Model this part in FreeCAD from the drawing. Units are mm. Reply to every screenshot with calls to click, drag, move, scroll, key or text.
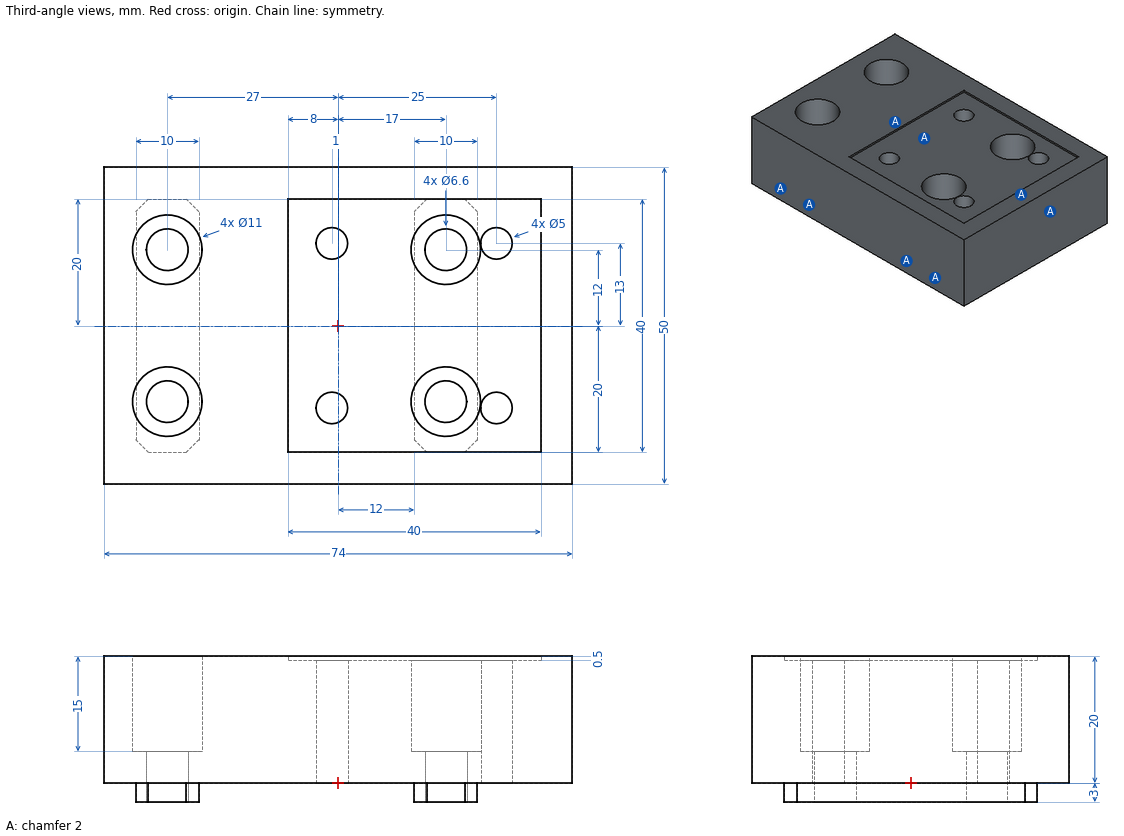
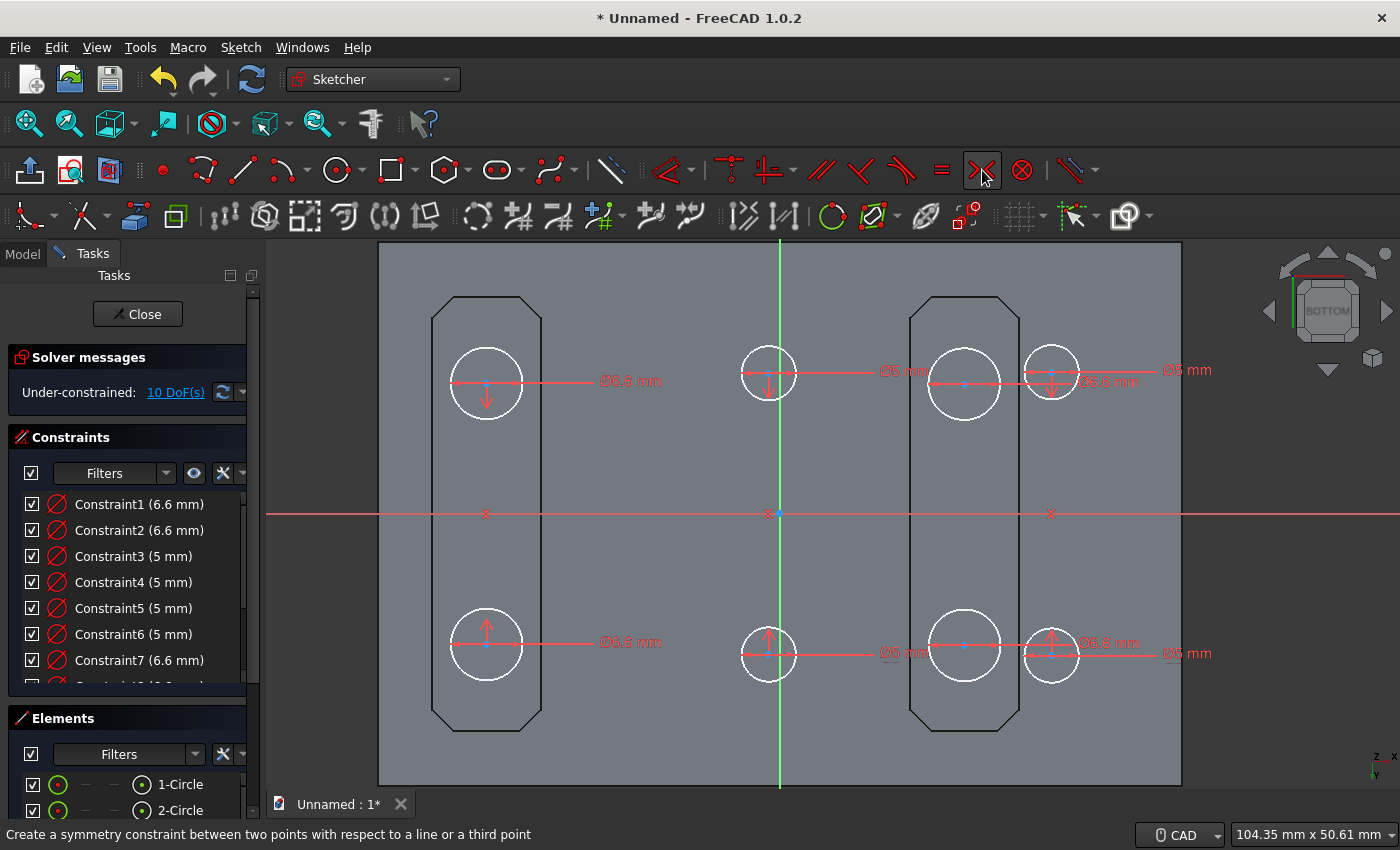
click(965, 645)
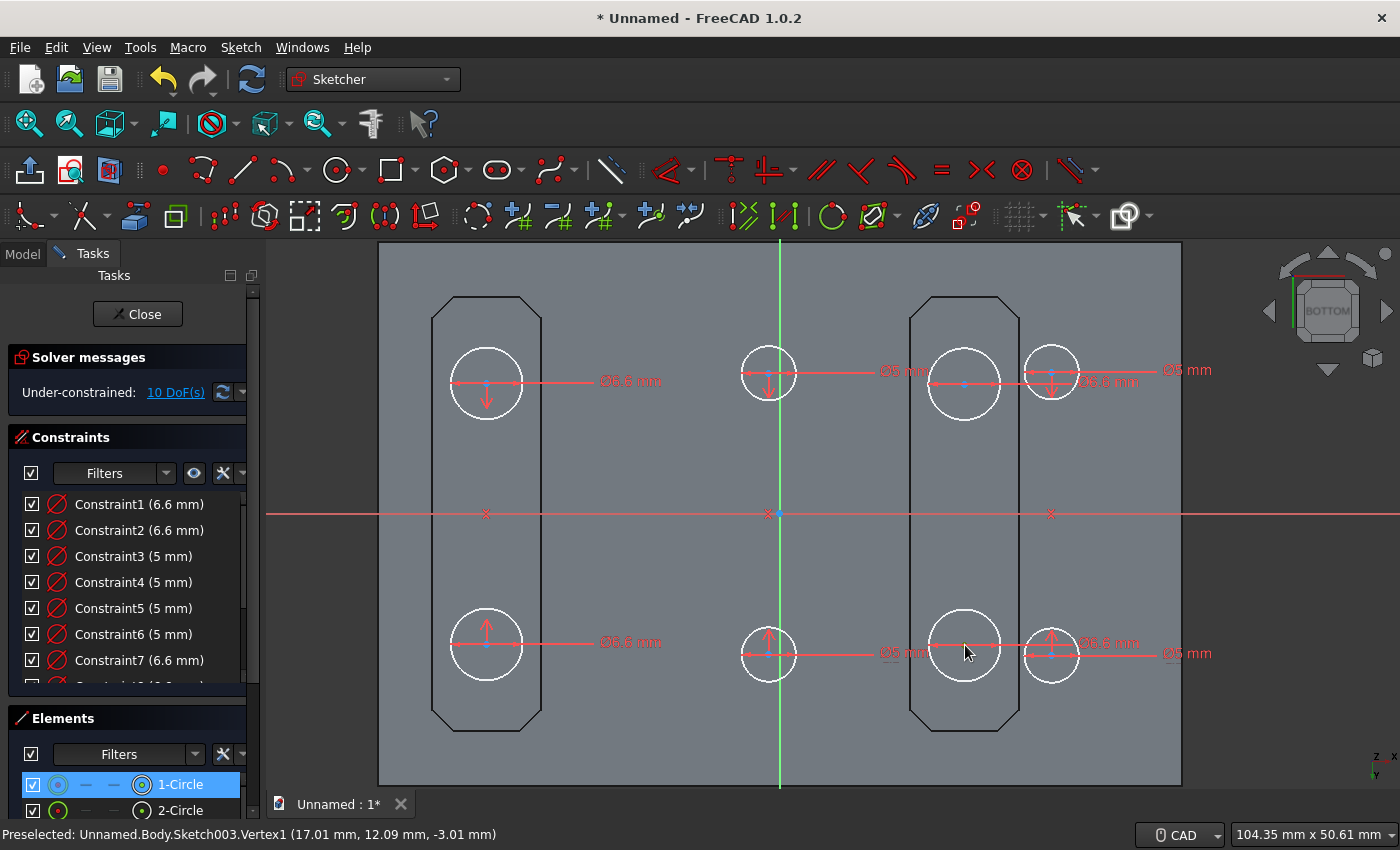
click(964, 384)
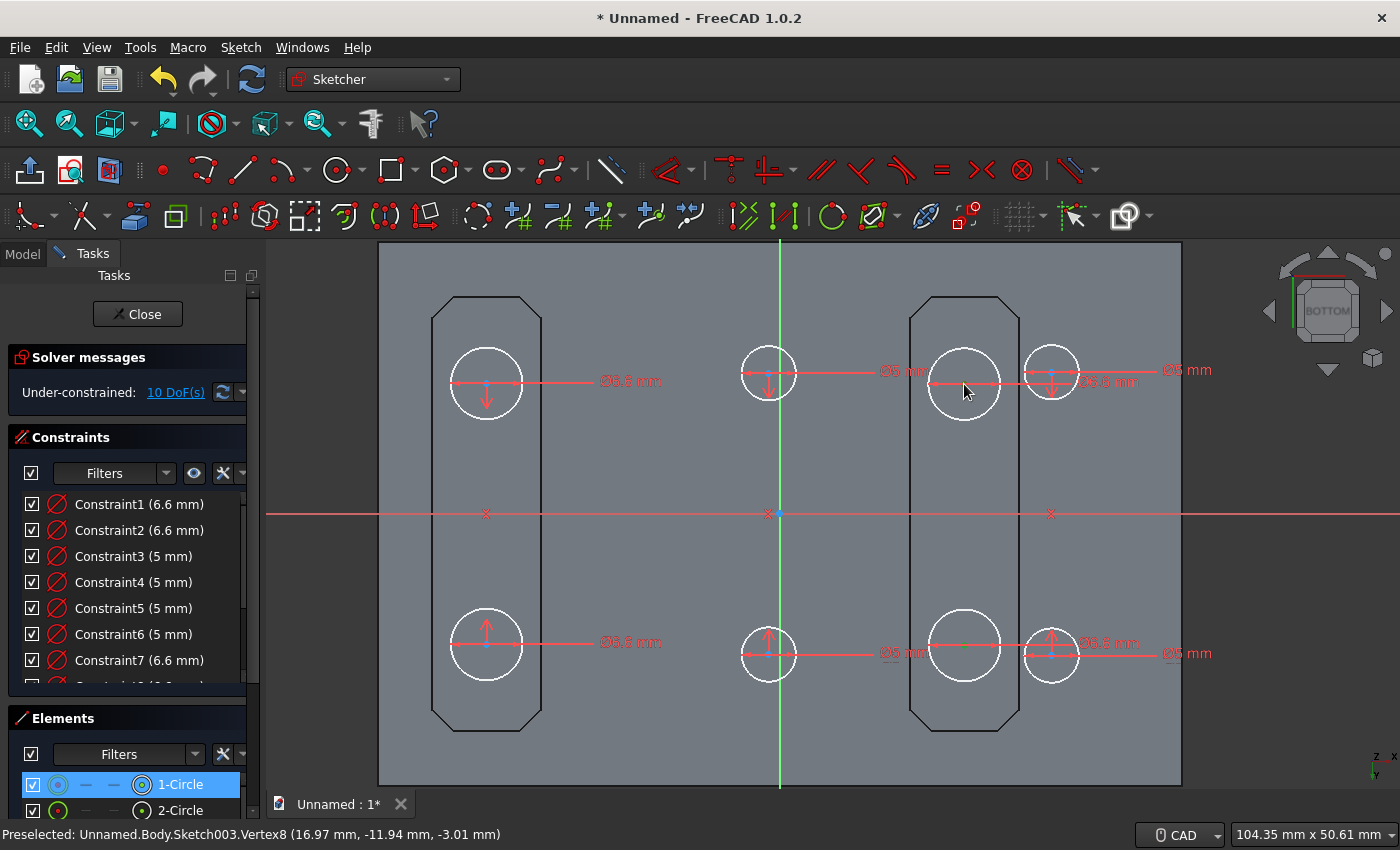
click(361, 514)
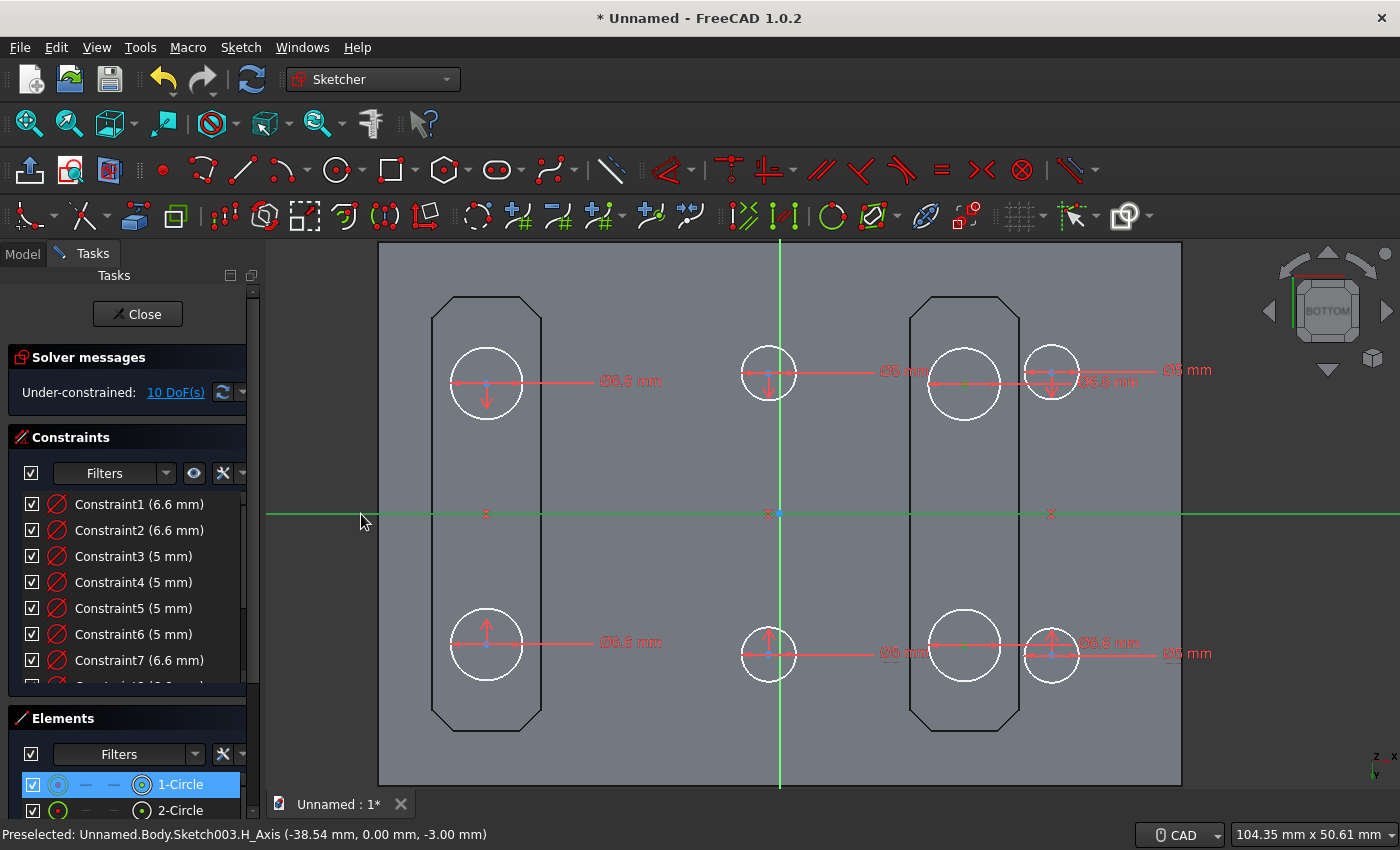
click(982, 170)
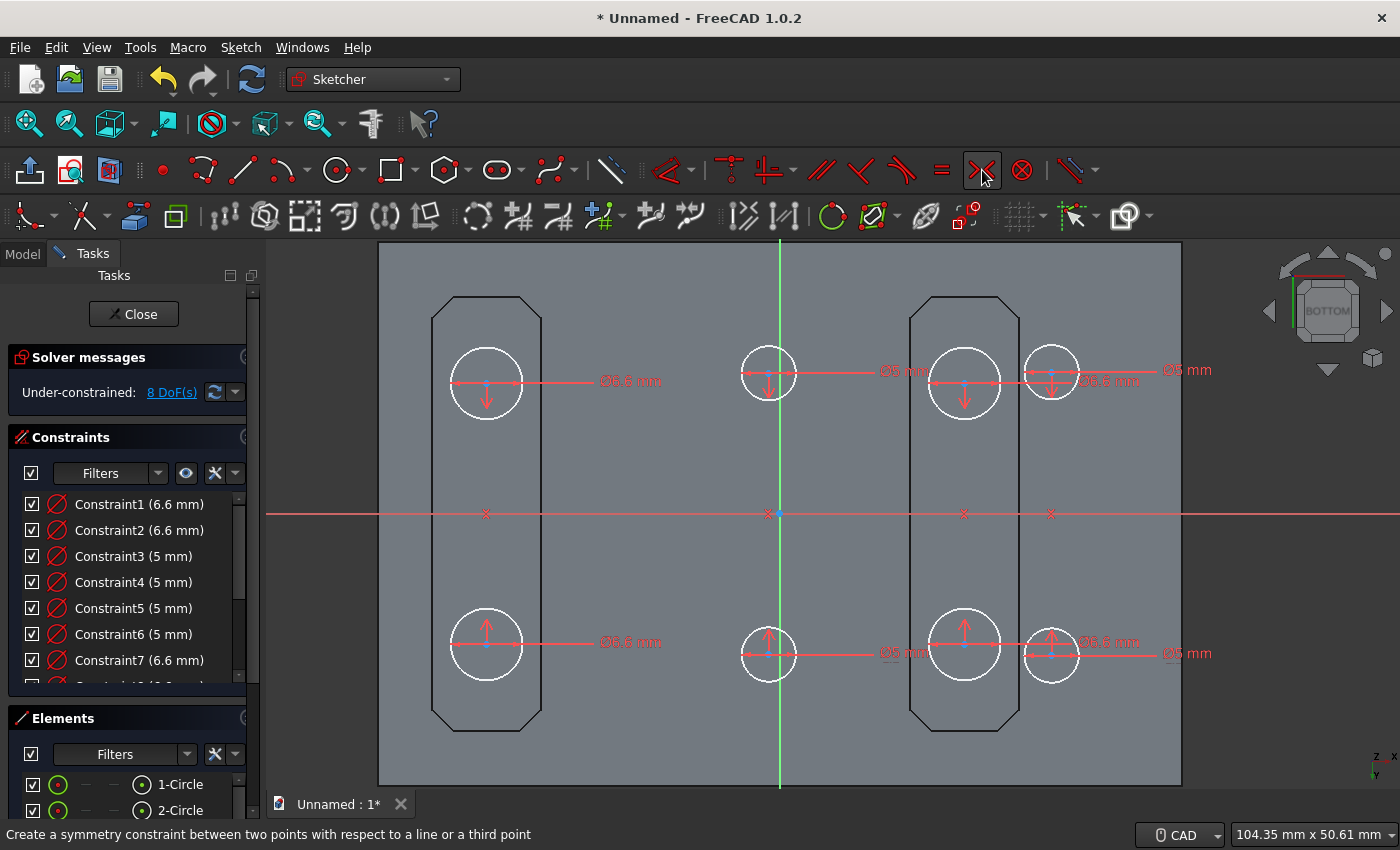
click(666, 170)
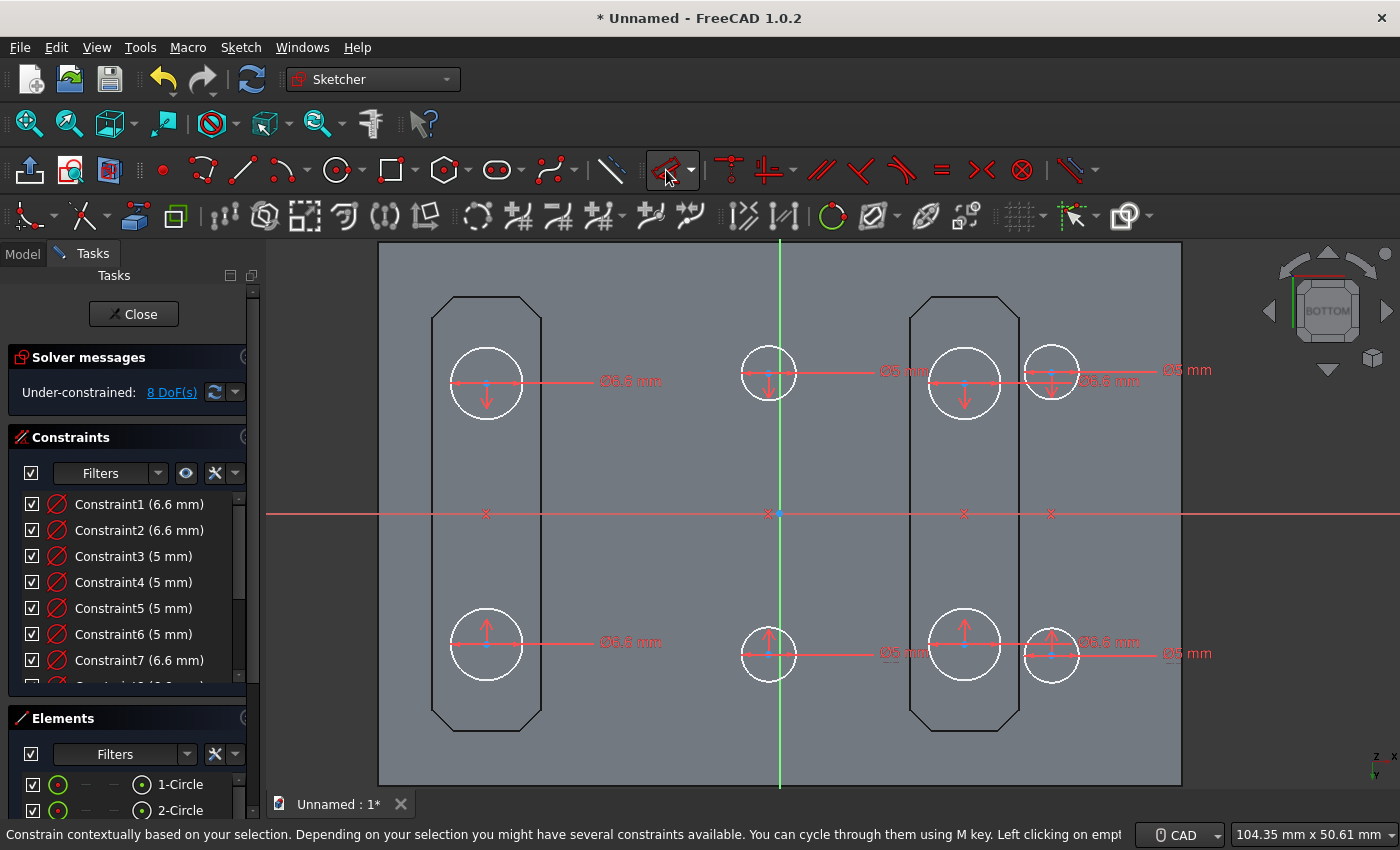
scroll(769, 655, up, 7)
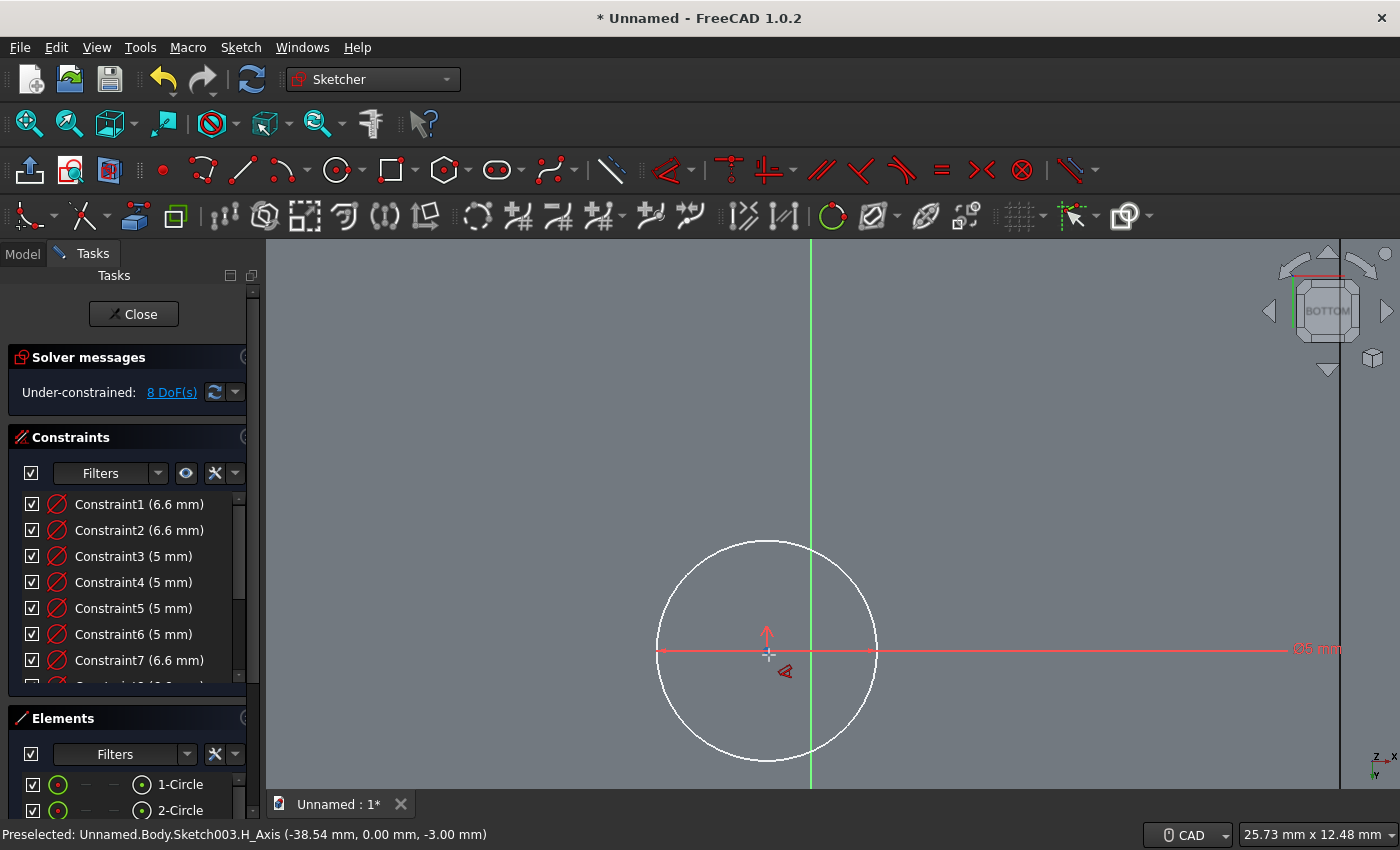
click(767, 651)
click(789, 685)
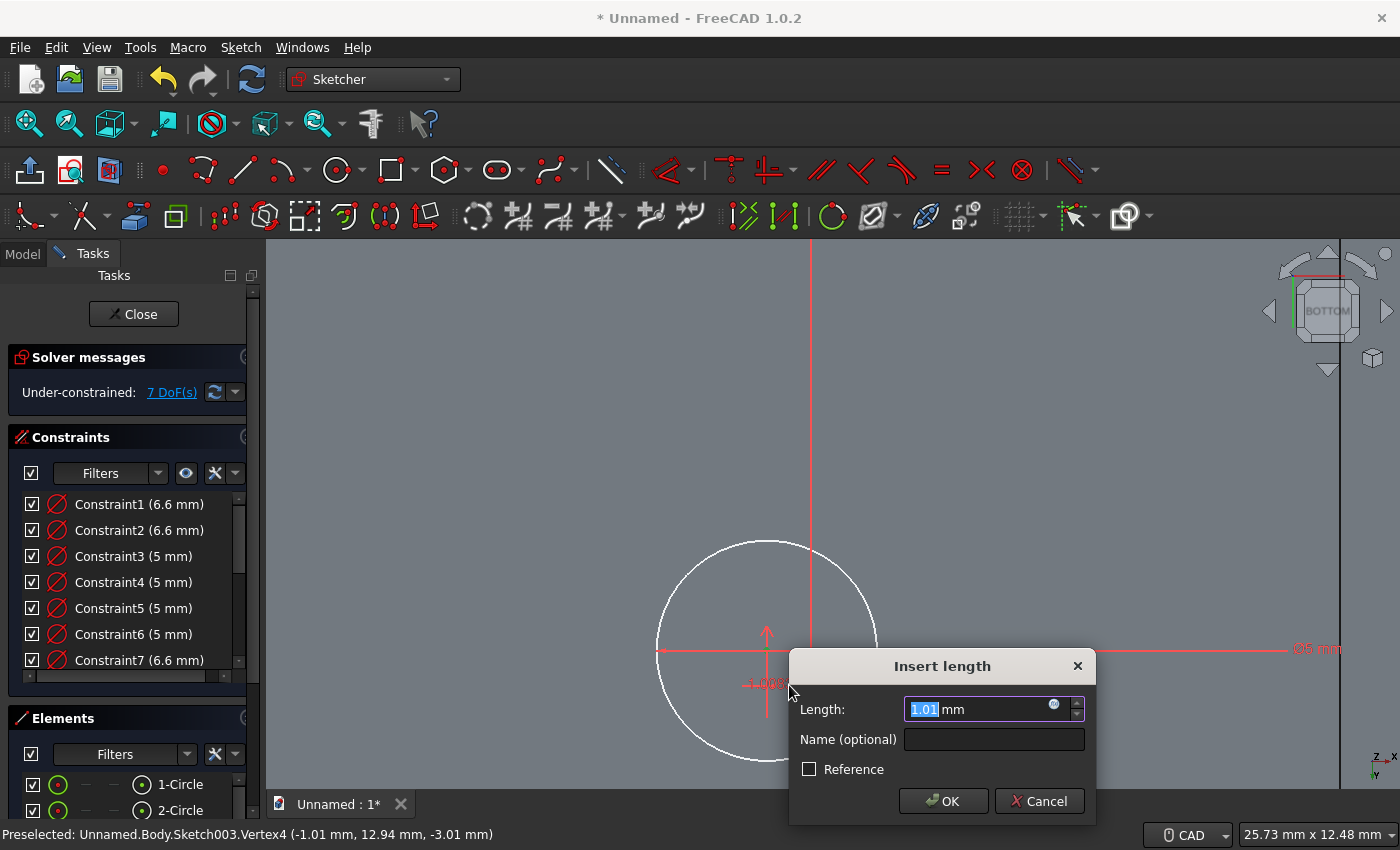
text(1)
key(Return)